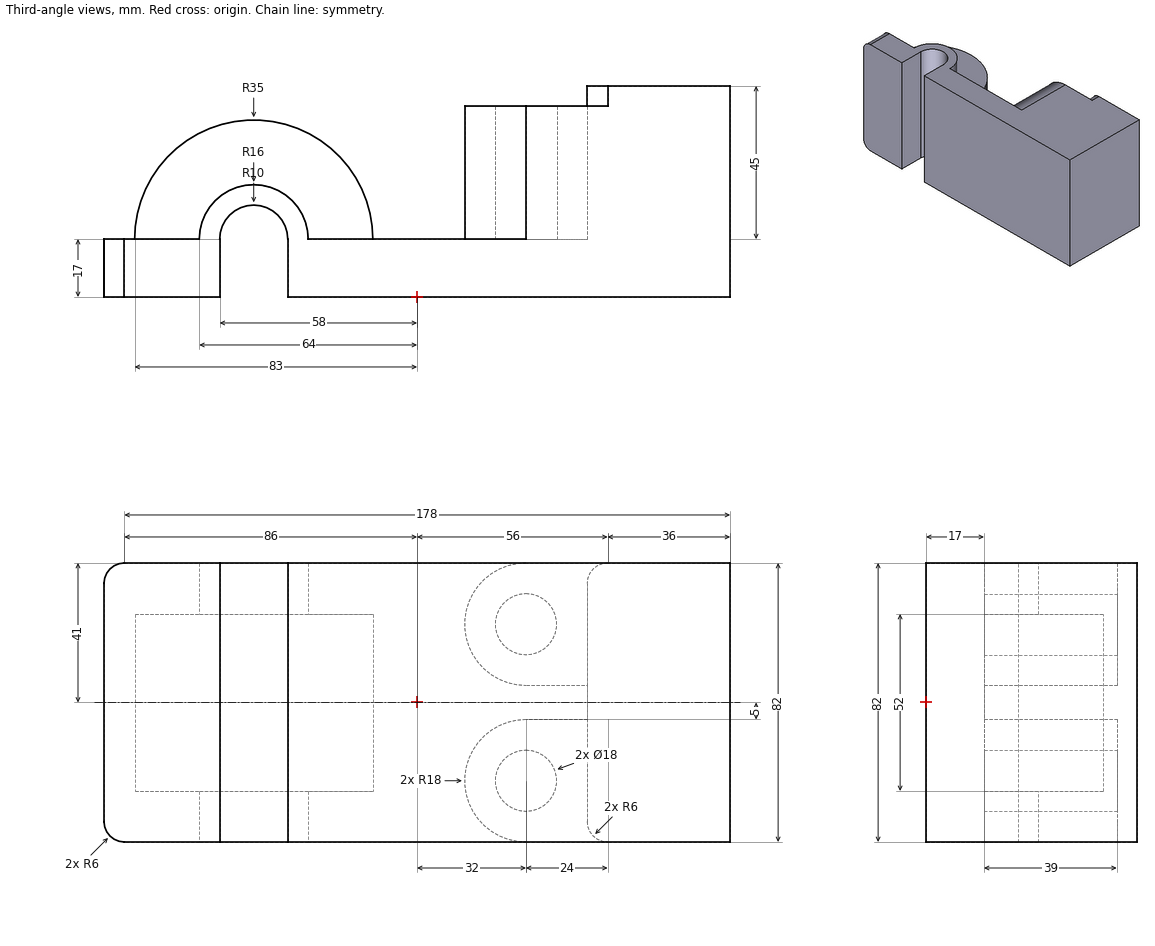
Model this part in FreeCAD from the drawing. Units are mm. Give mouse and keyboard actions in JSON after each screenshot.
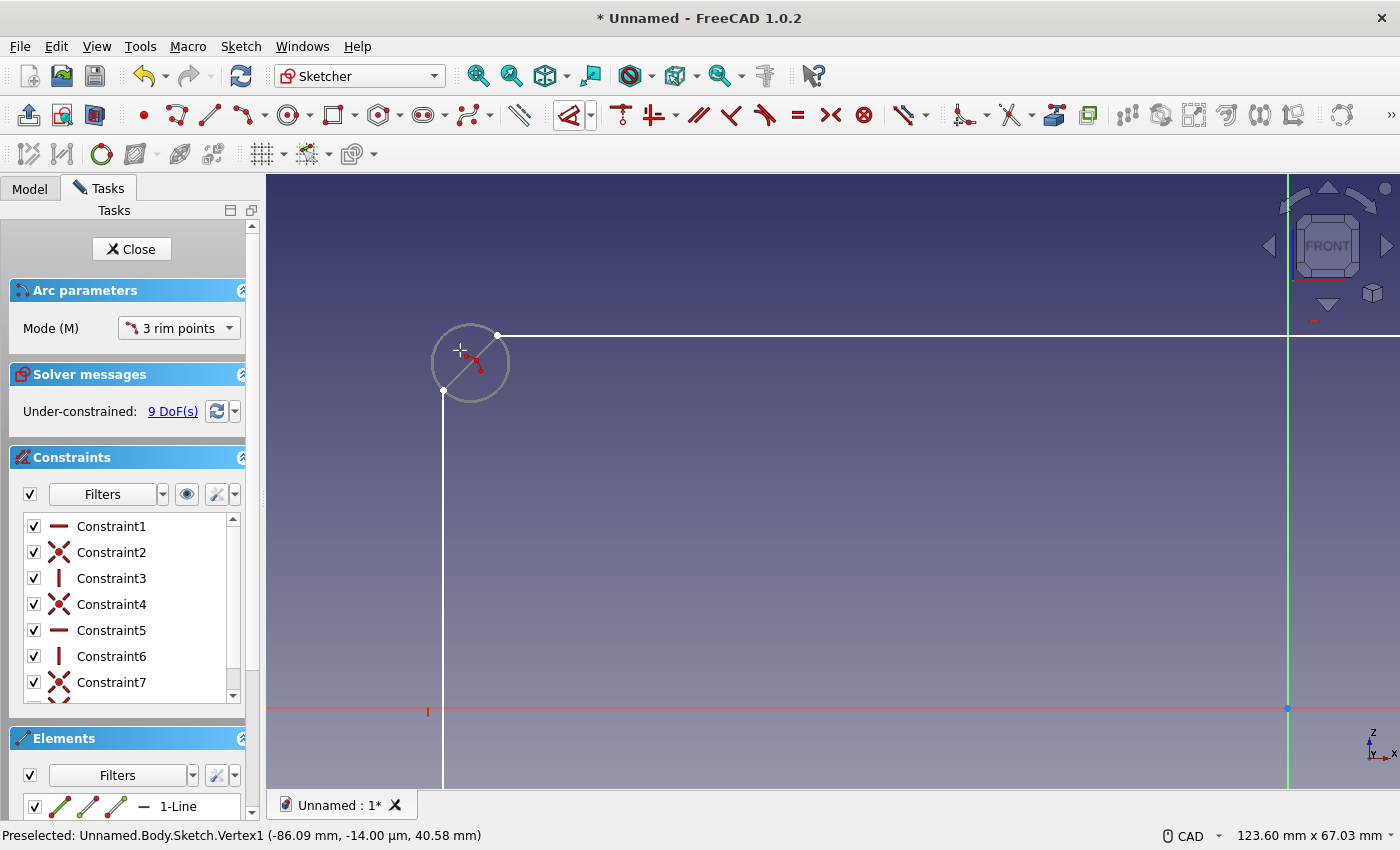
{"action": "left_click", "coordinate": [460, 348]}
{"action": "key", "text": "Escape"}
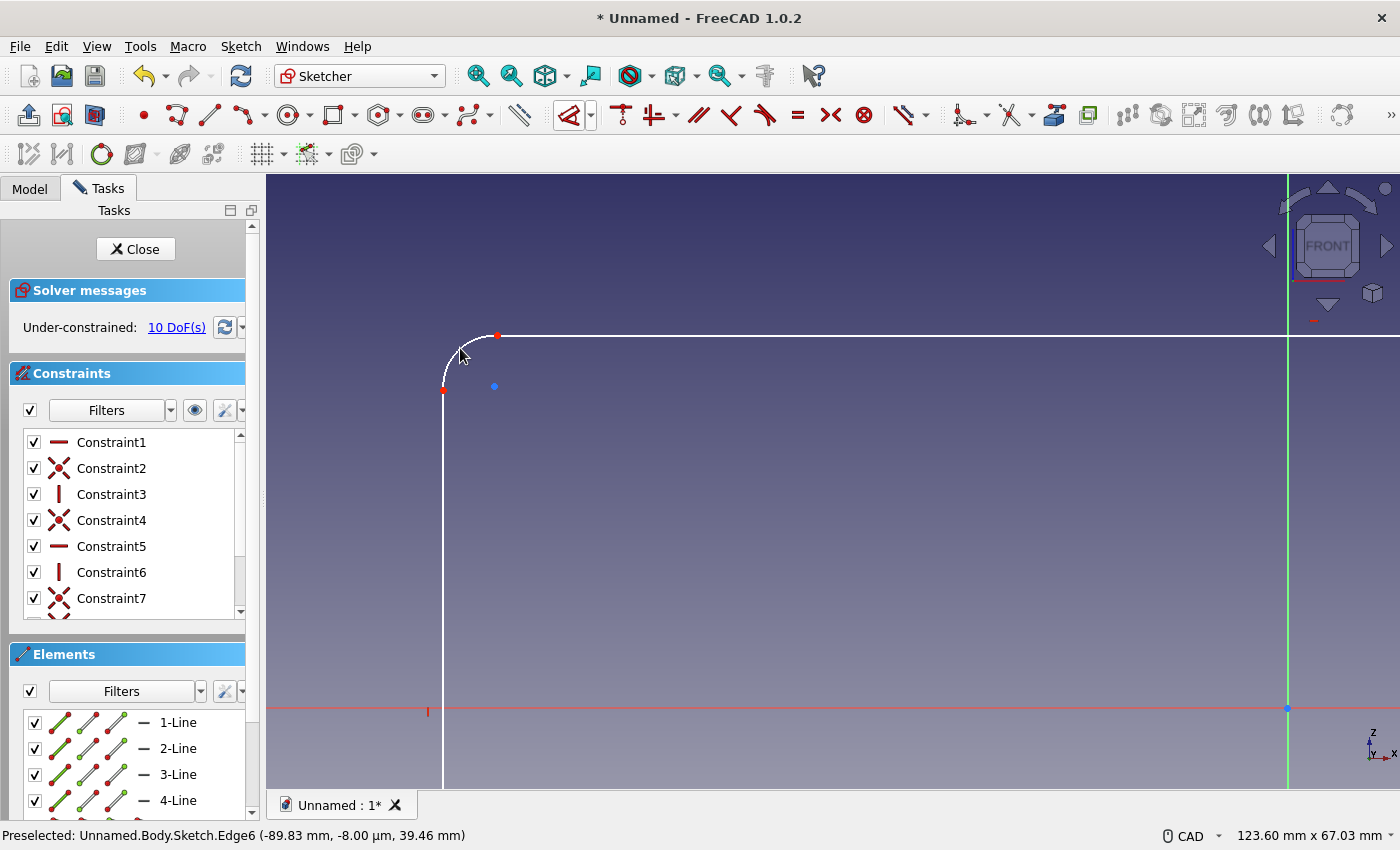
{"action": "left_click", "coordinate": [988, 336]}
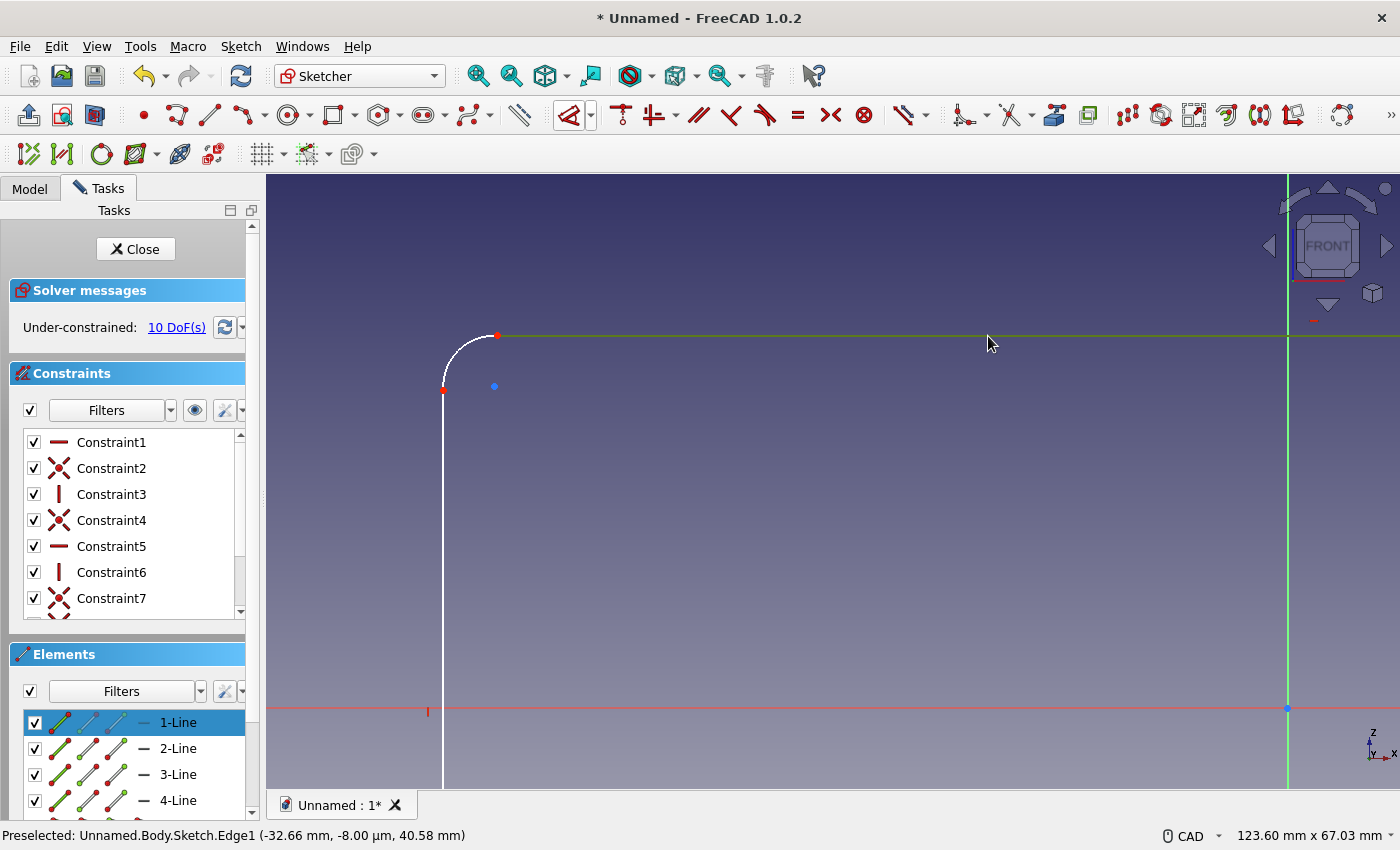
{"action": "left_click", "coordinate": [472, 341]}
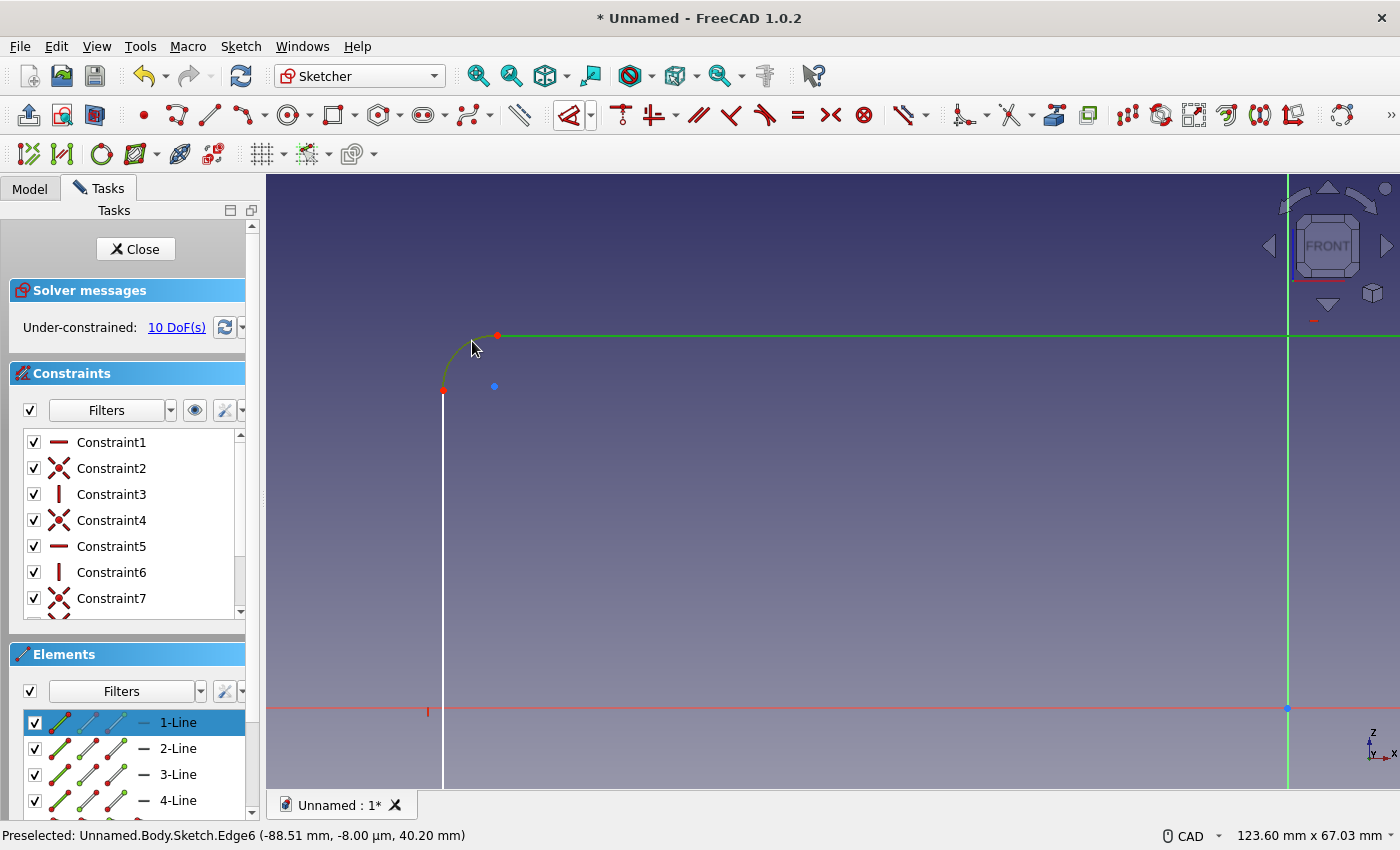
{"action": "left_click", "coordinate": [765, 116]}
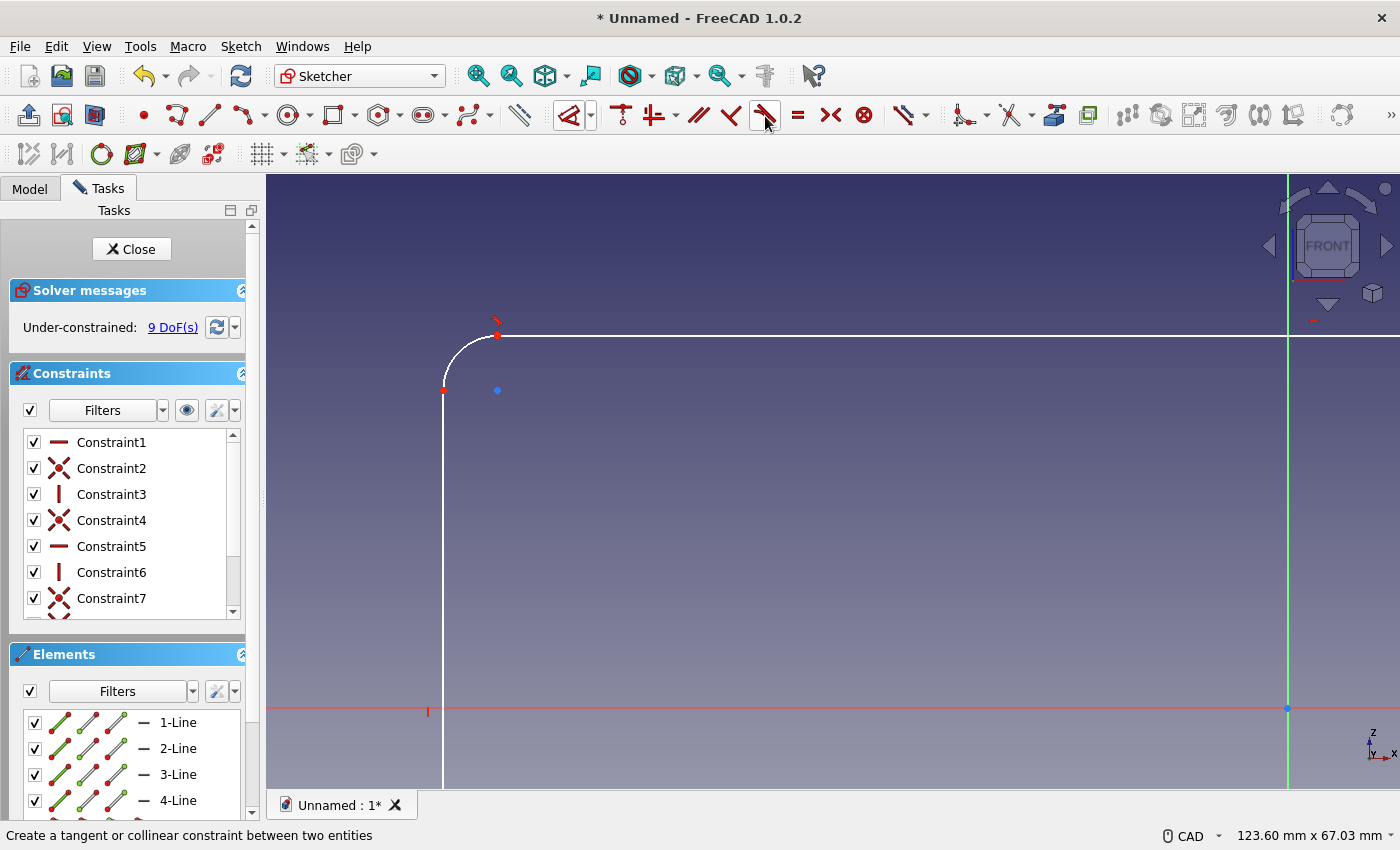
{"action": "scroll", "coordinate": [460, 350], "scroll_direction": "down", "scroll_amount": 5}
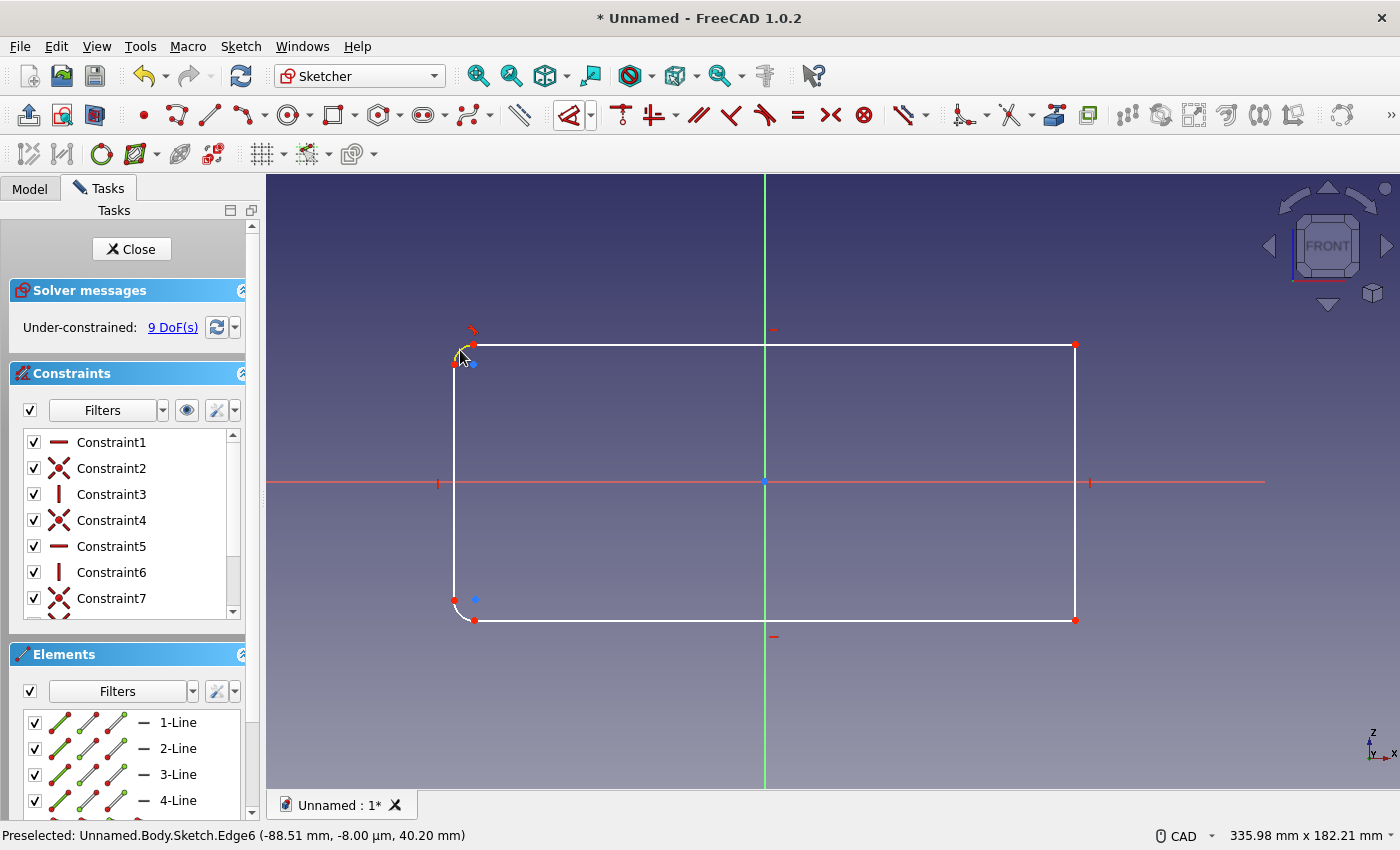
{"action": "left_click", "coordinate": [895, 621]}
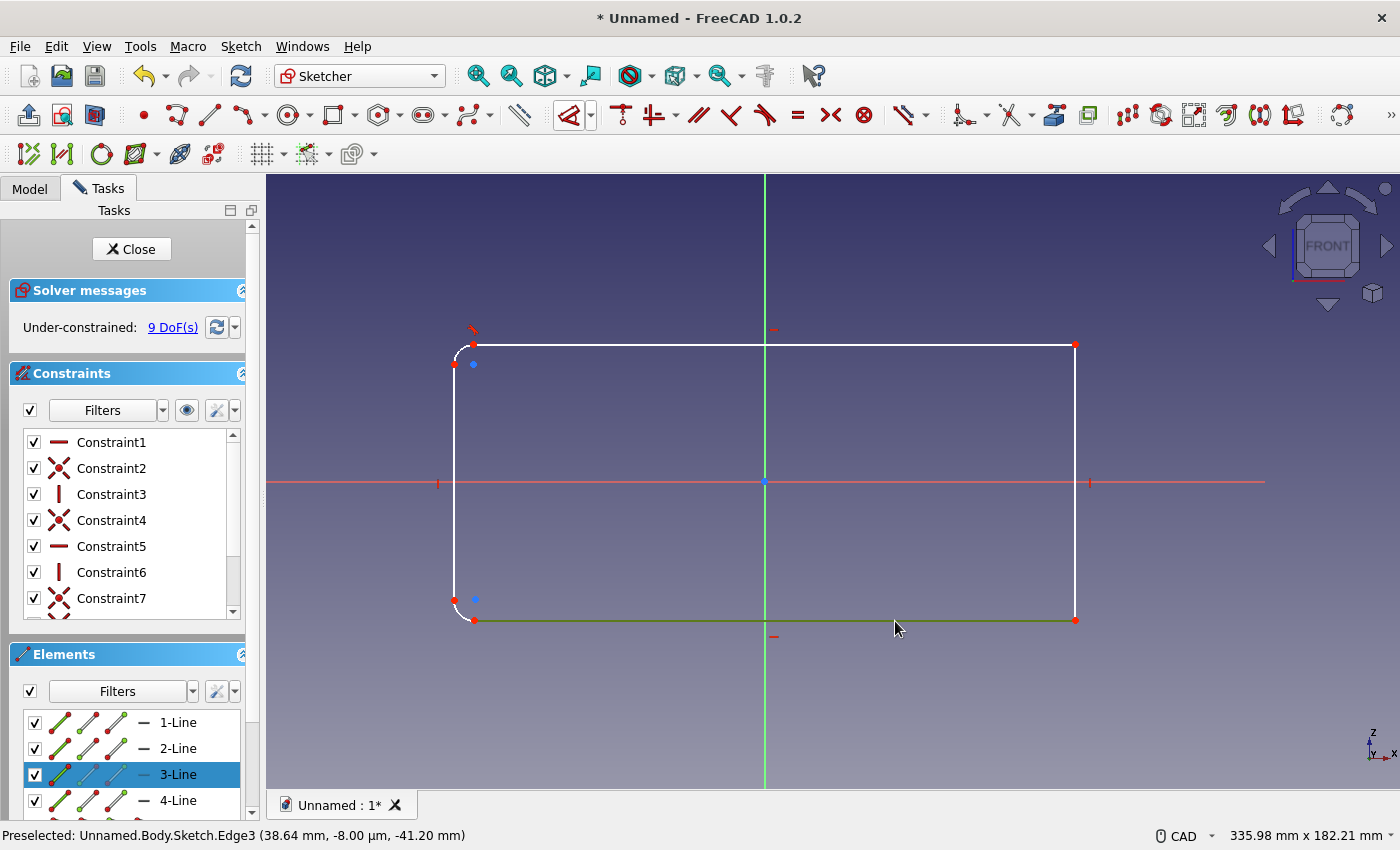
{"action": "scroll", "coordinate": [456, 610], "scroll_direction": "up", "scroll_amount": 3}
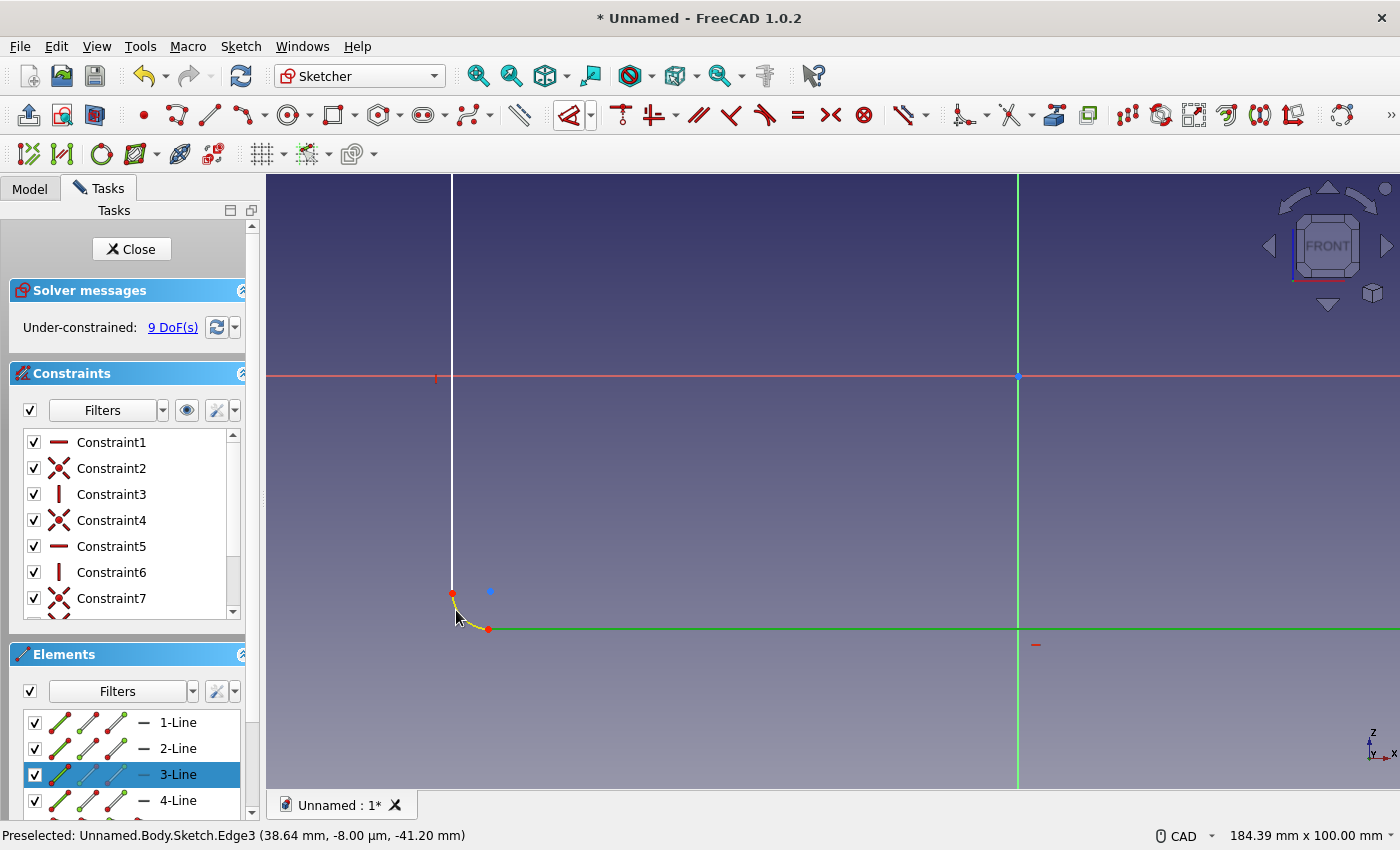
{"action": "left_click", "coordinate": [457, 609]}